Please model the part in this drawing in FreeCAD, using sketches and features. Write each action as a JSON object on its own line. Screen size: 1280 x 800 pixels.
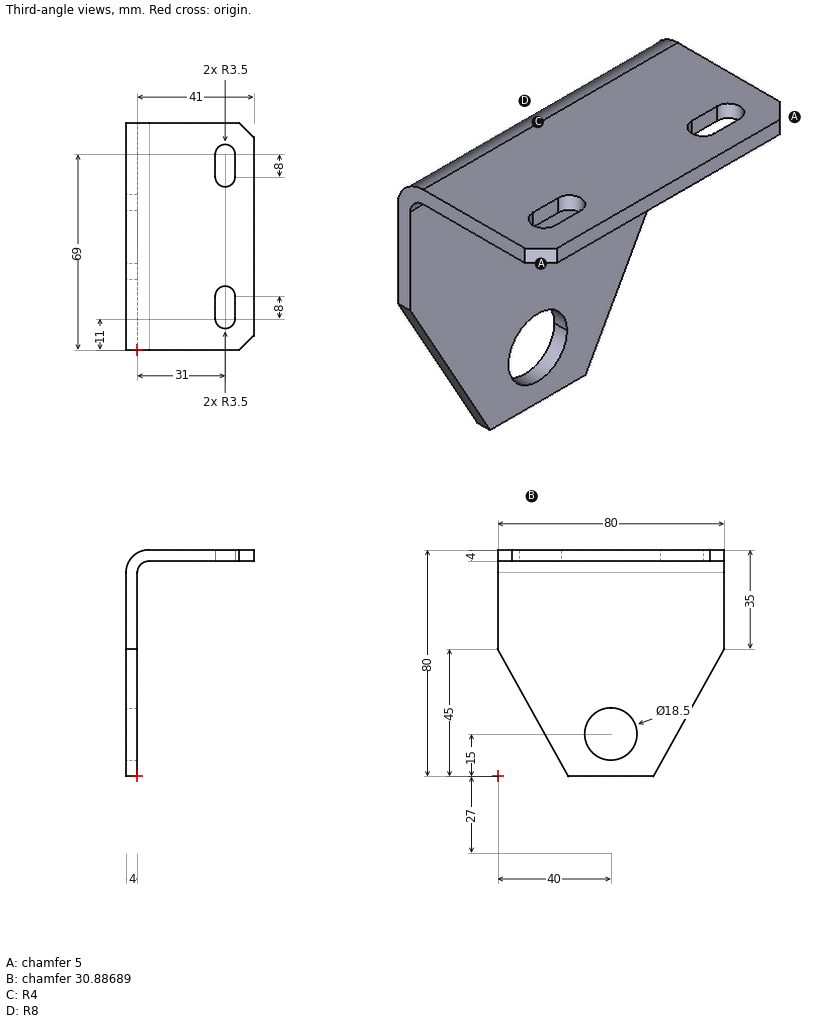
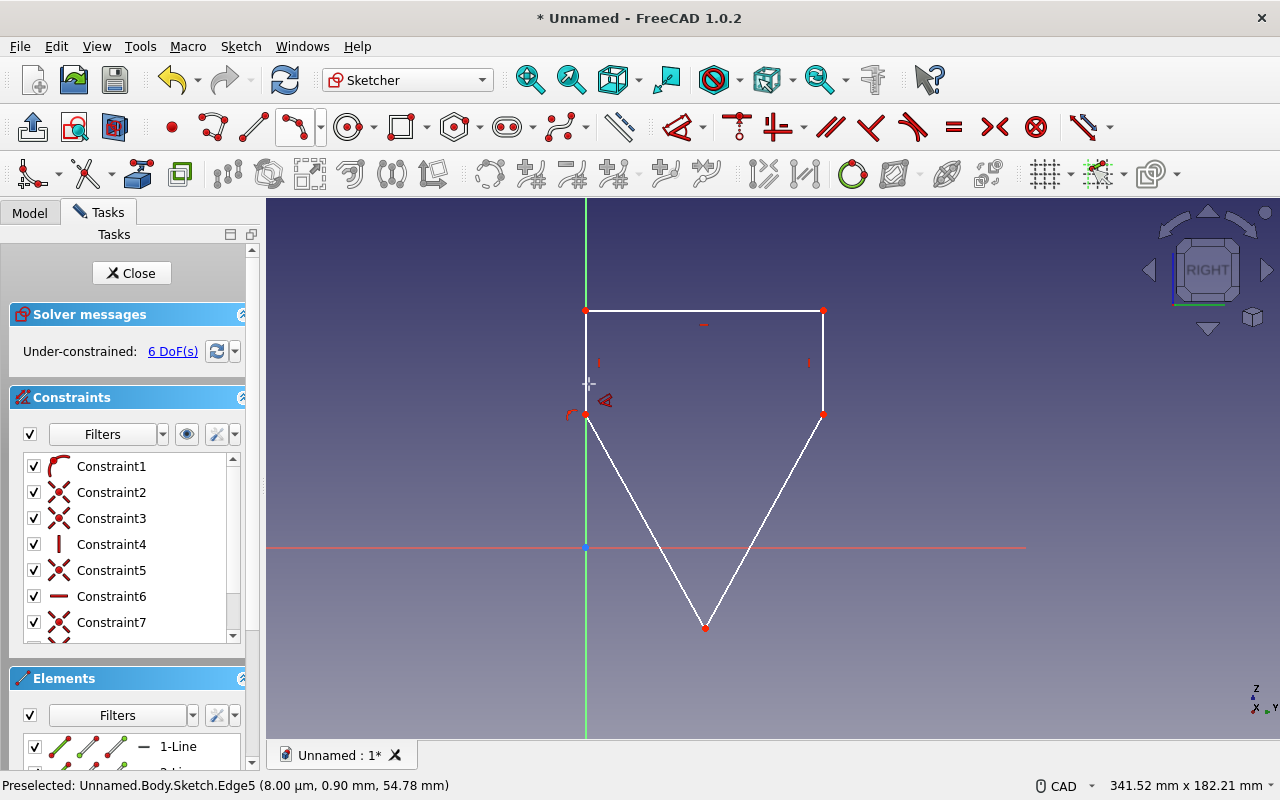
{"action": "left_click", "coordinate": [823, 384]}
{"action": "left_click", "coordinate": [857, 363]}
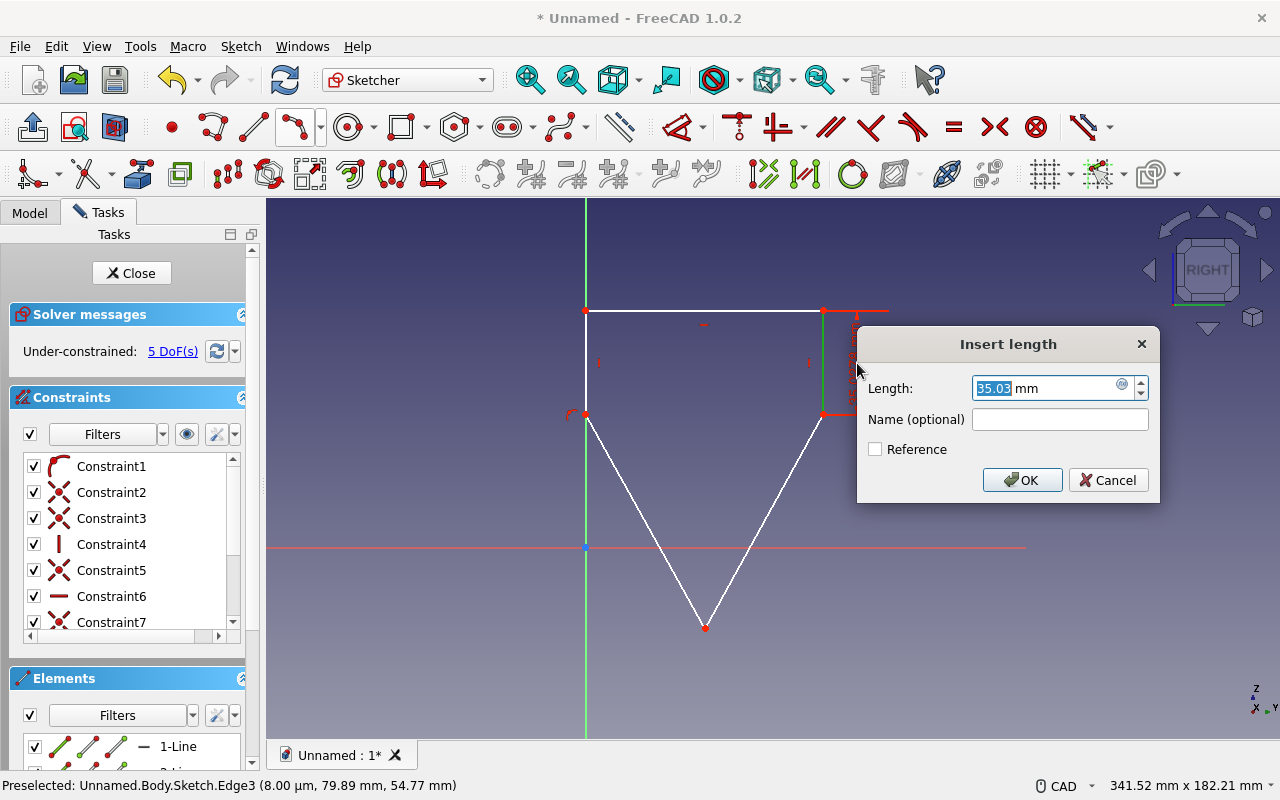
{"action": "type", "text": "35"}
{"action": "key", "text": "Return"}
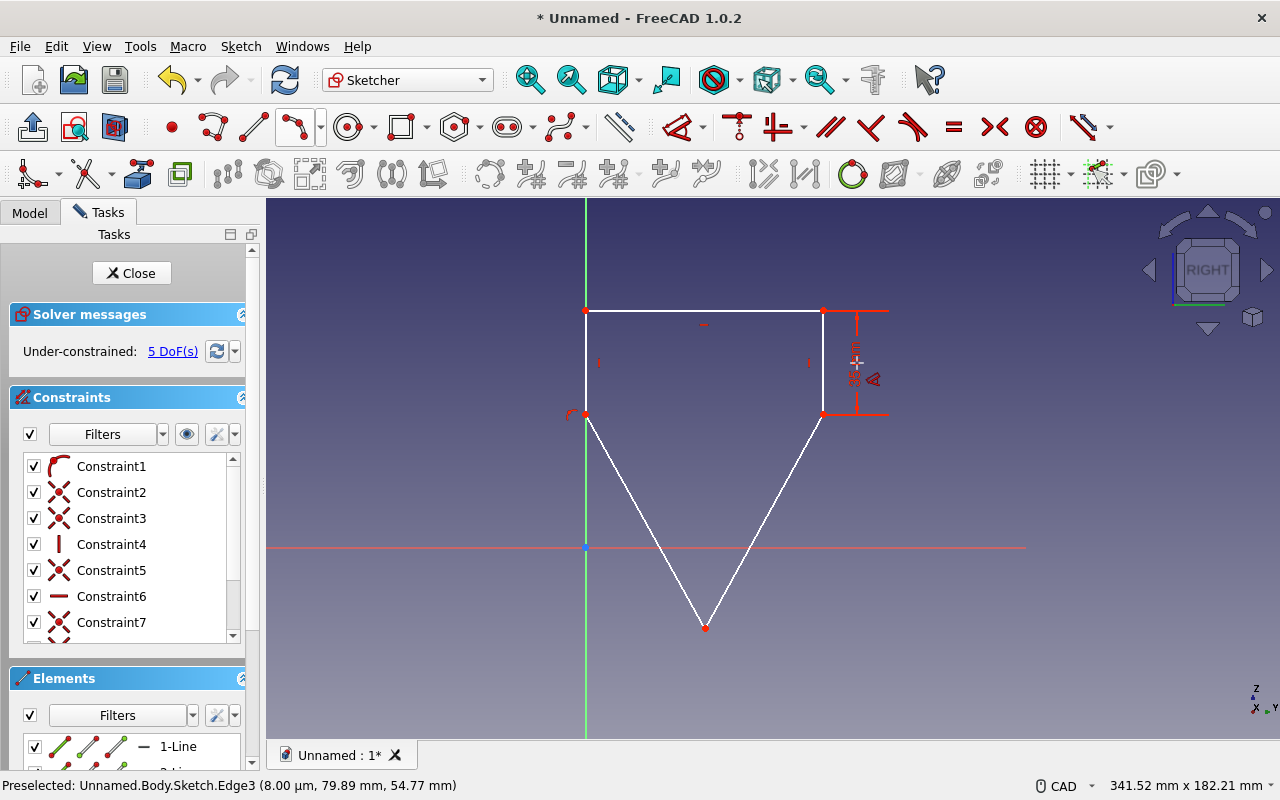
{"action": "left_click", "coordinate": [752, 311]}
{"action": "left_click", "coordinate": [704, 277]}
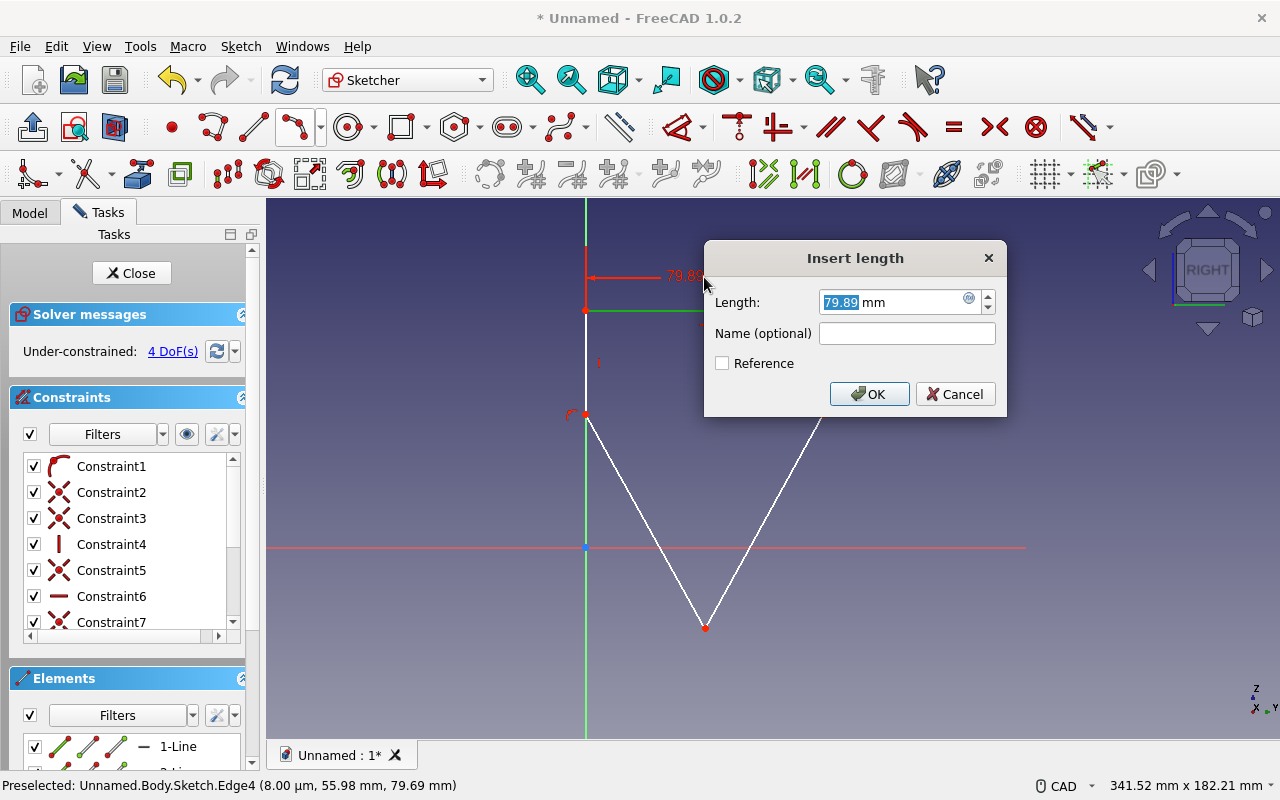
{"action": "type", "text": "80"}
{"action": "key", "text": "Return"}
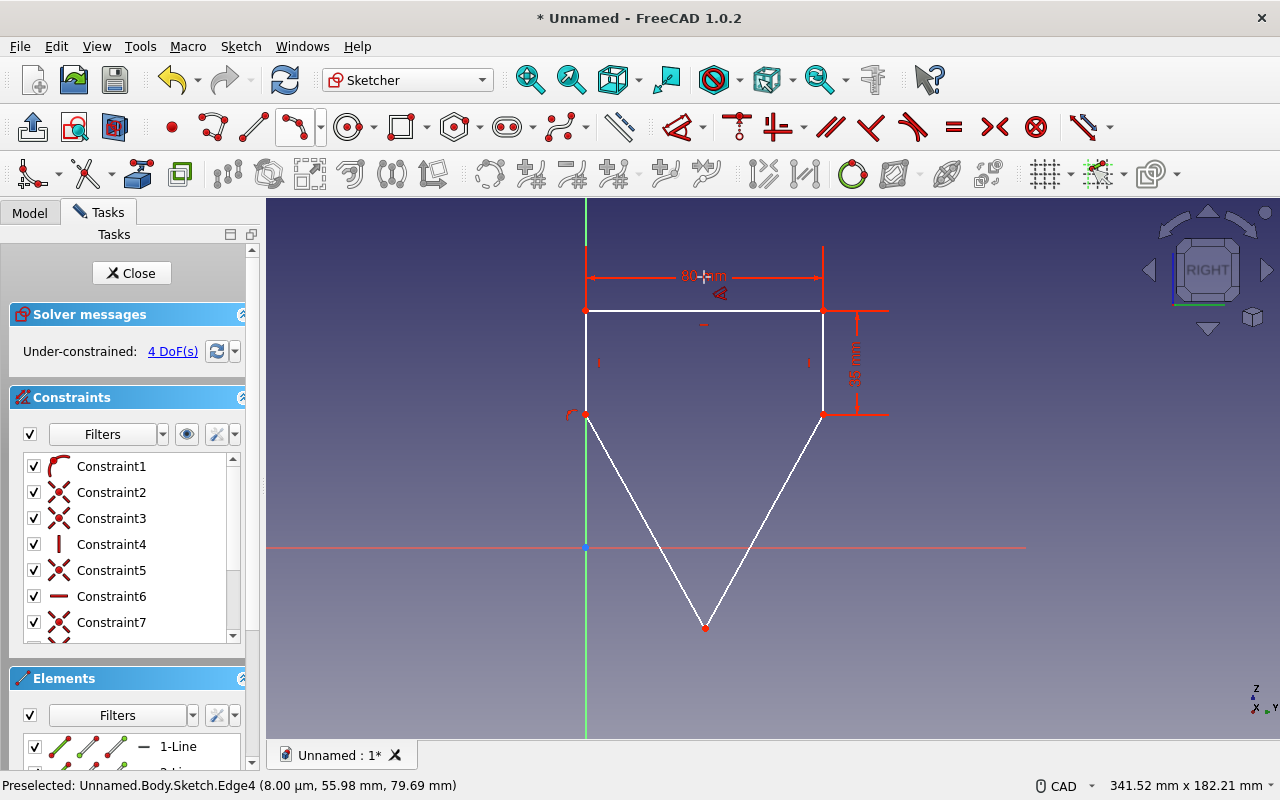
{"action": "left_click", "coordinate": [586, 342]}
{"action": "left_click", "coordinate": [552, 363]}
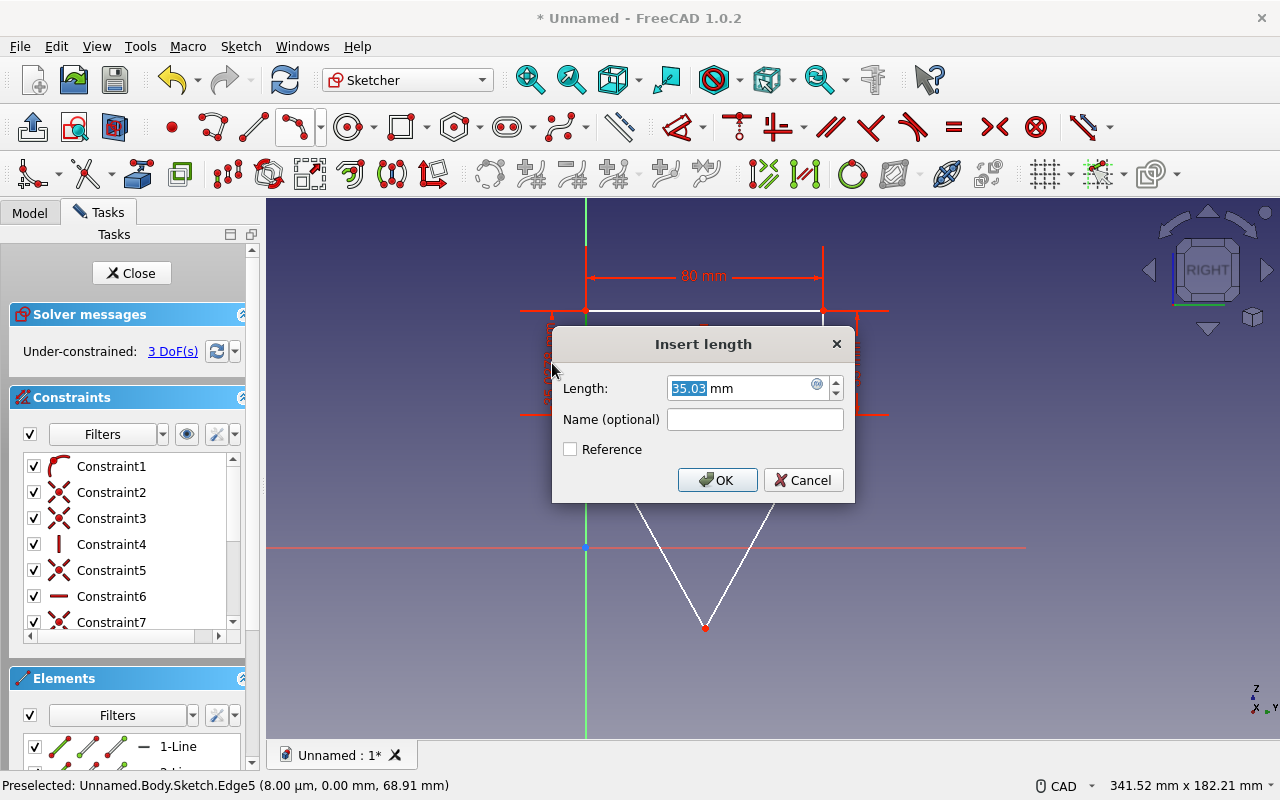
{"action": "type", "text": "35"}
{"action": "key", "text": "Return"}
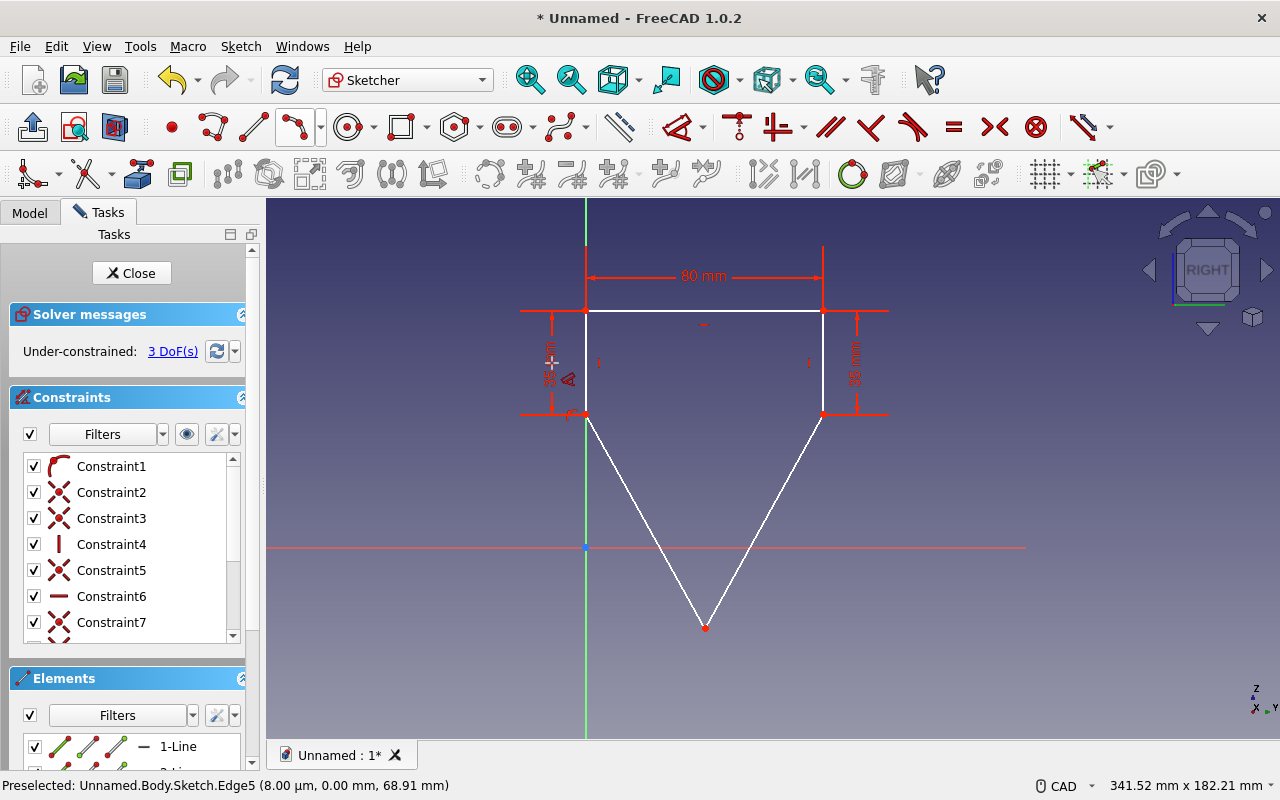
{"action": "left_click", "coordinate": [586, 415]}
{"action": "left_click", "coordinate": [552, 481]}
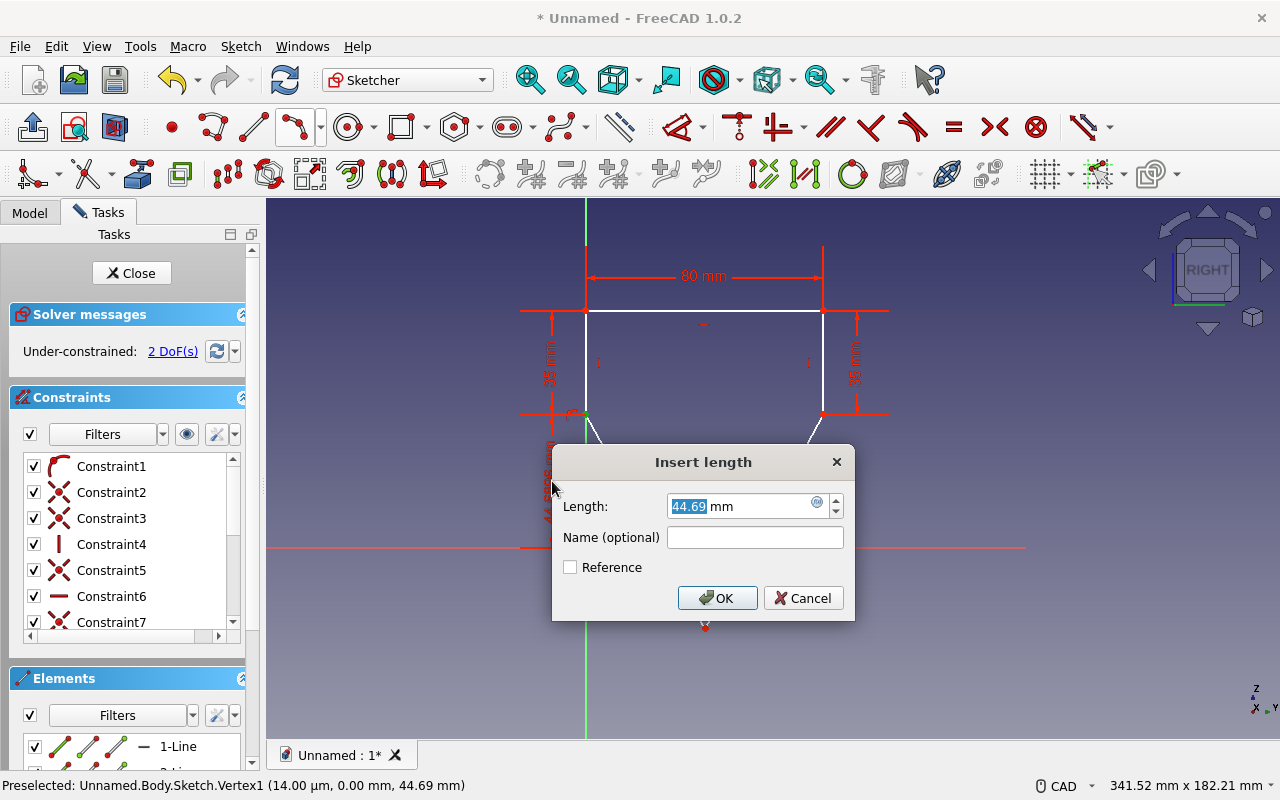
{"action": "type", "text": "45"}
{"action": "key", "text": "Return"}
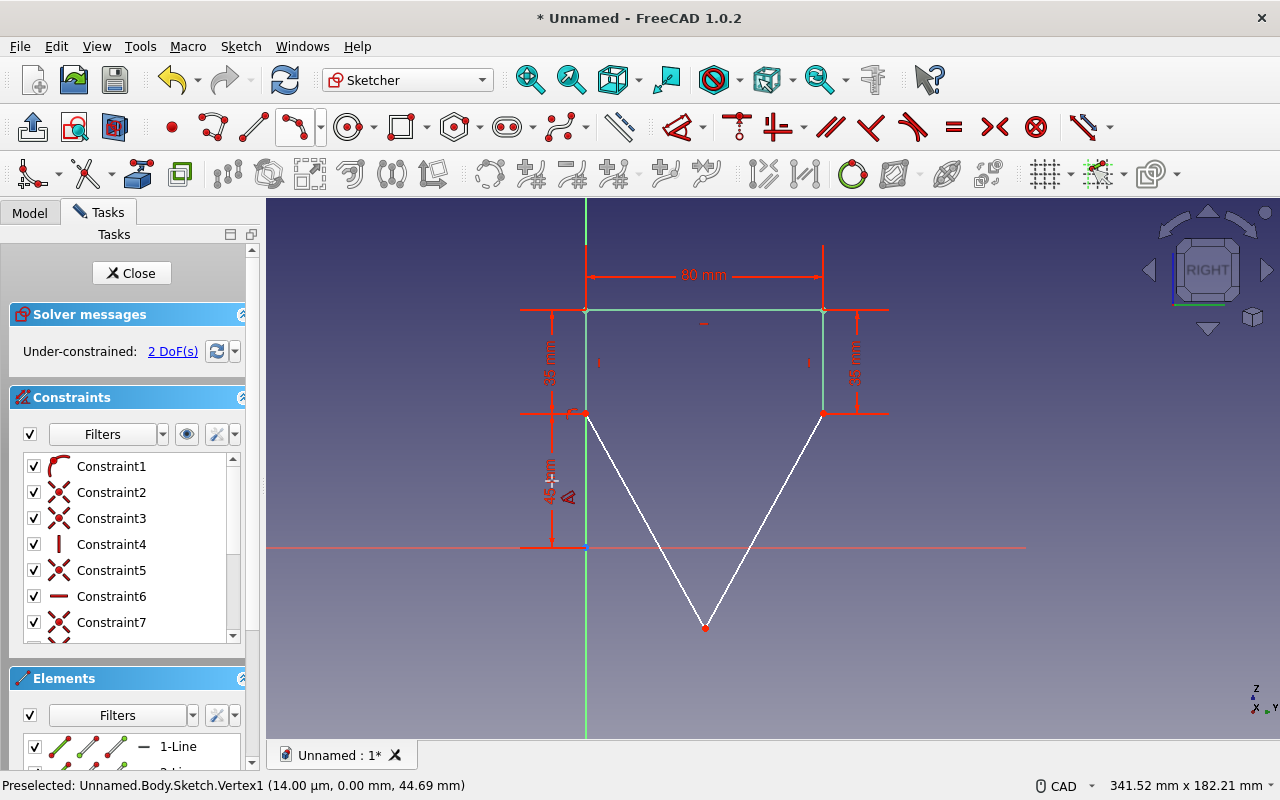
{"action": "left_click", "coordinate": [705, 629]}
{"action": "left_click", "coordinate": [645, 663]}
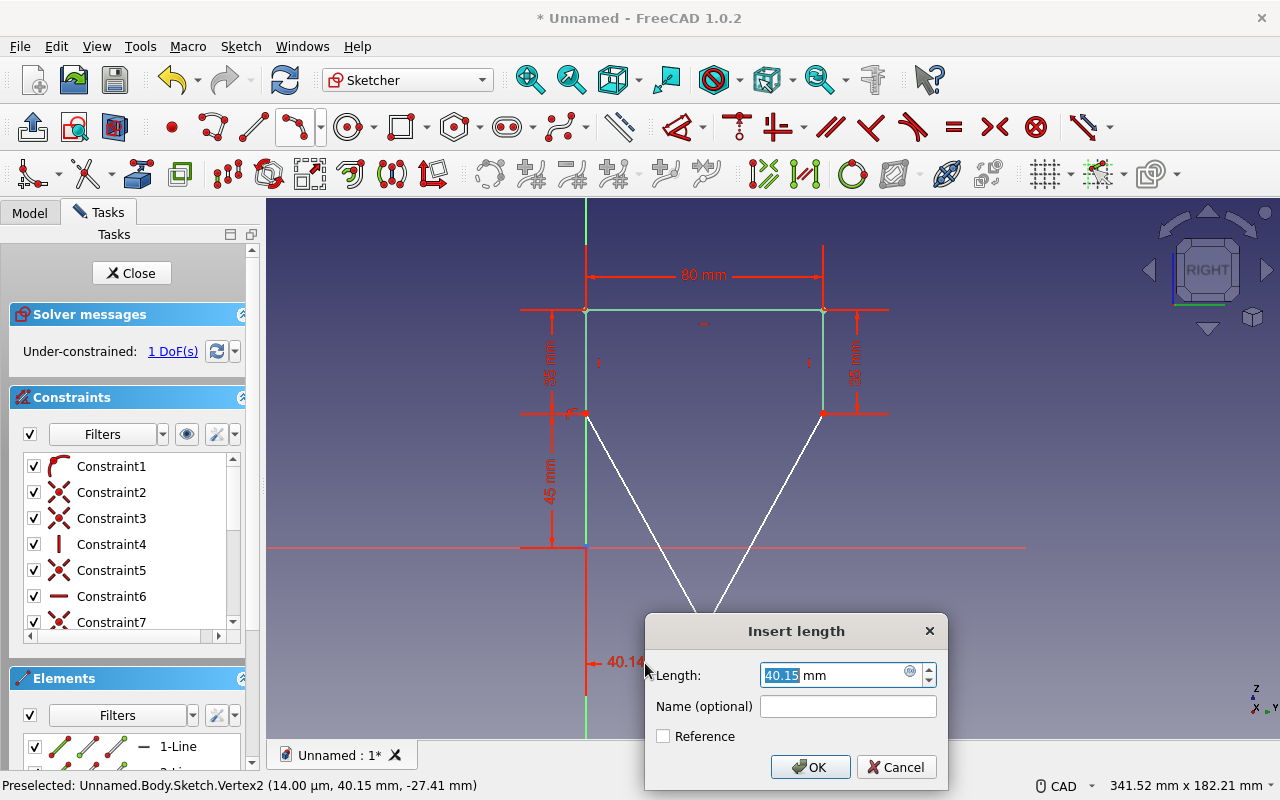
{"action": "type", "text": "40"}
{"action": "key", "text": "Return"}